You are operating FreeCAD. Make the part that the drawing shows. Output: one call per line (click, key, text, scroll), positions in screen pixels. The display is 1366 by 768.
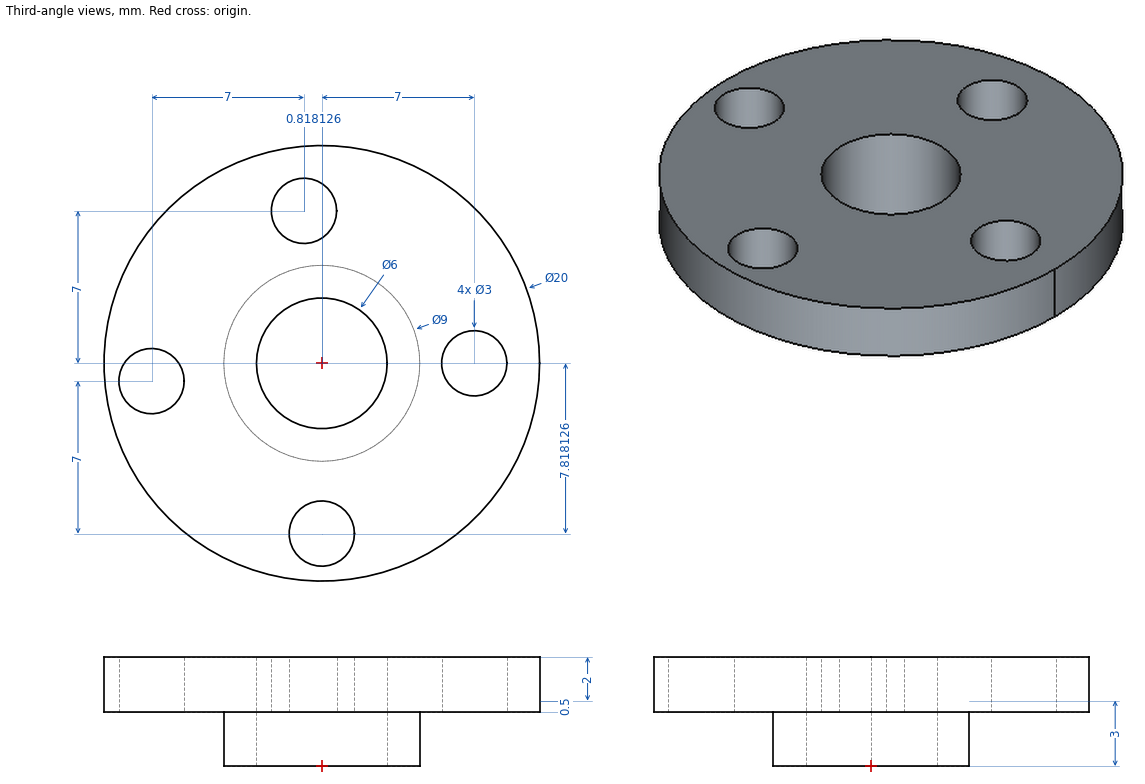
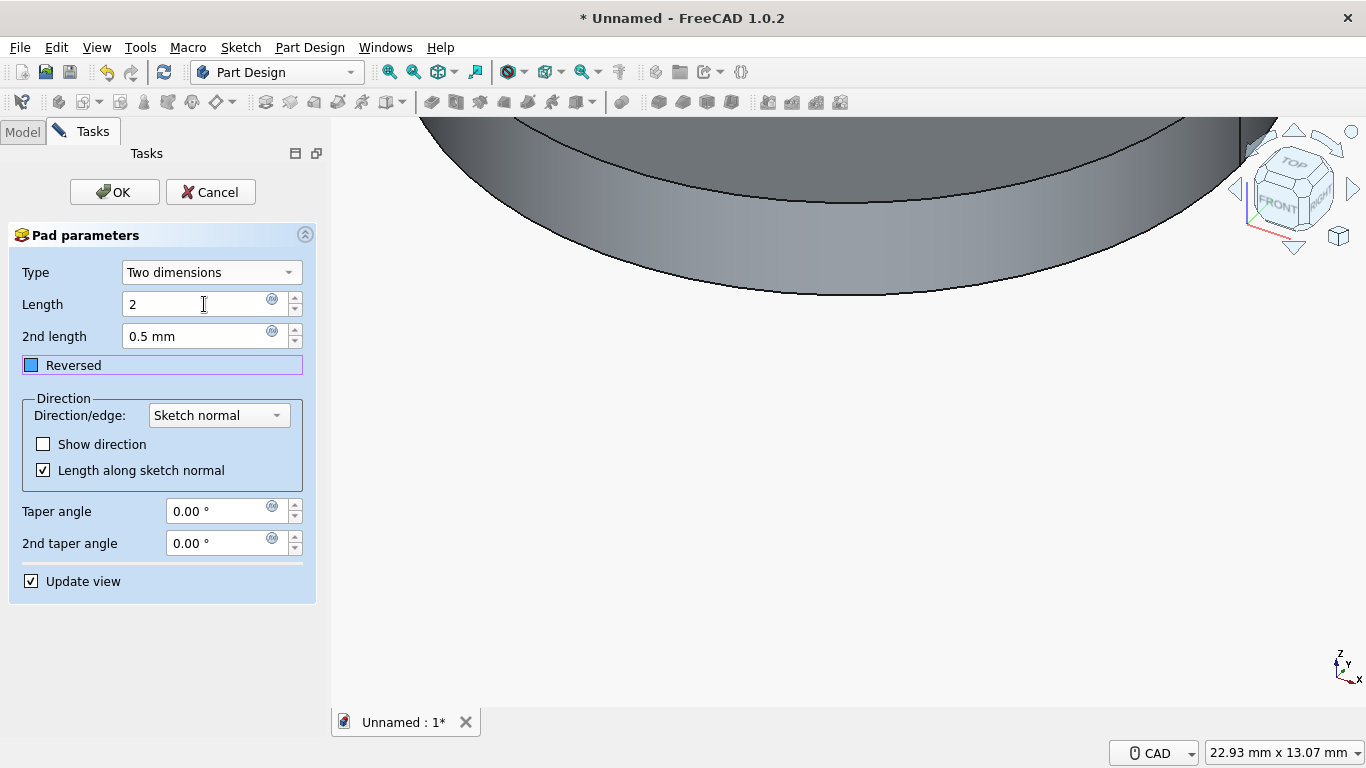
click(115, 192)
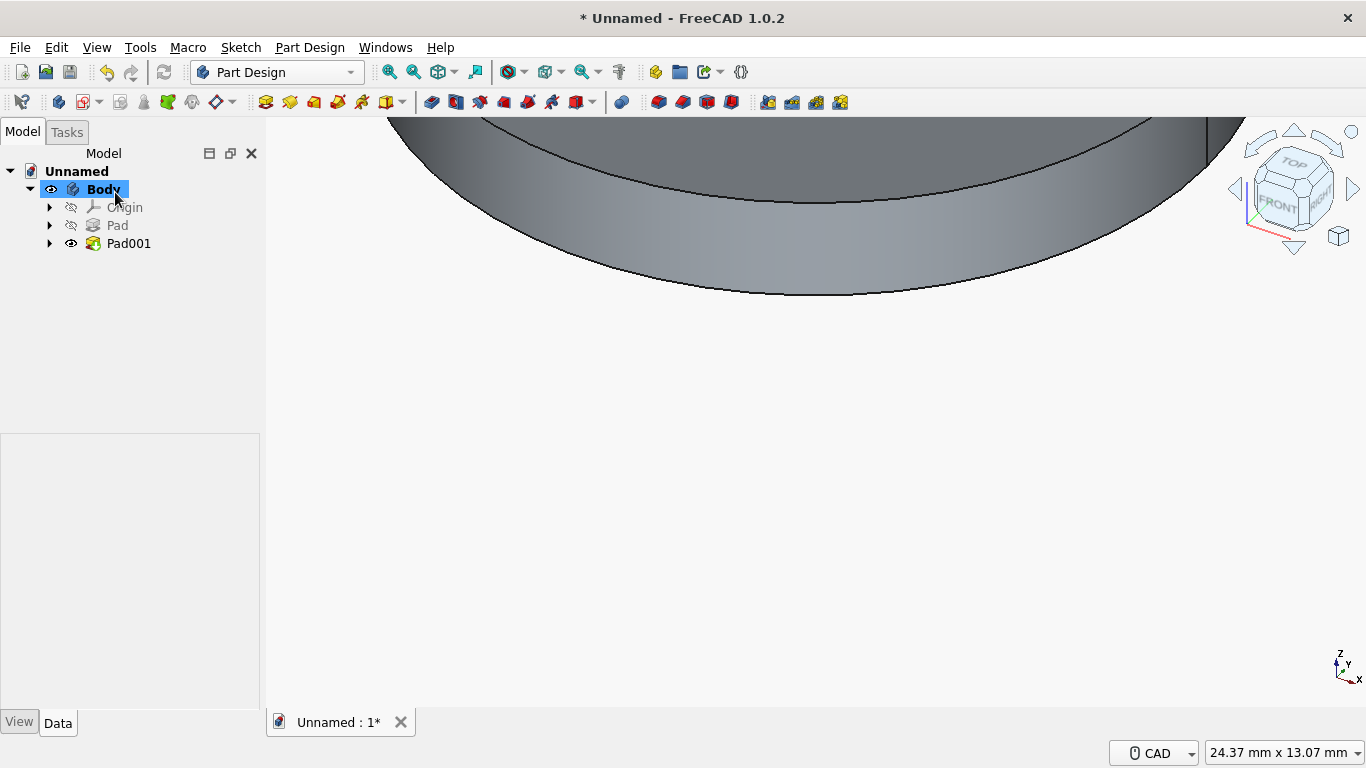
key(v)
key(f)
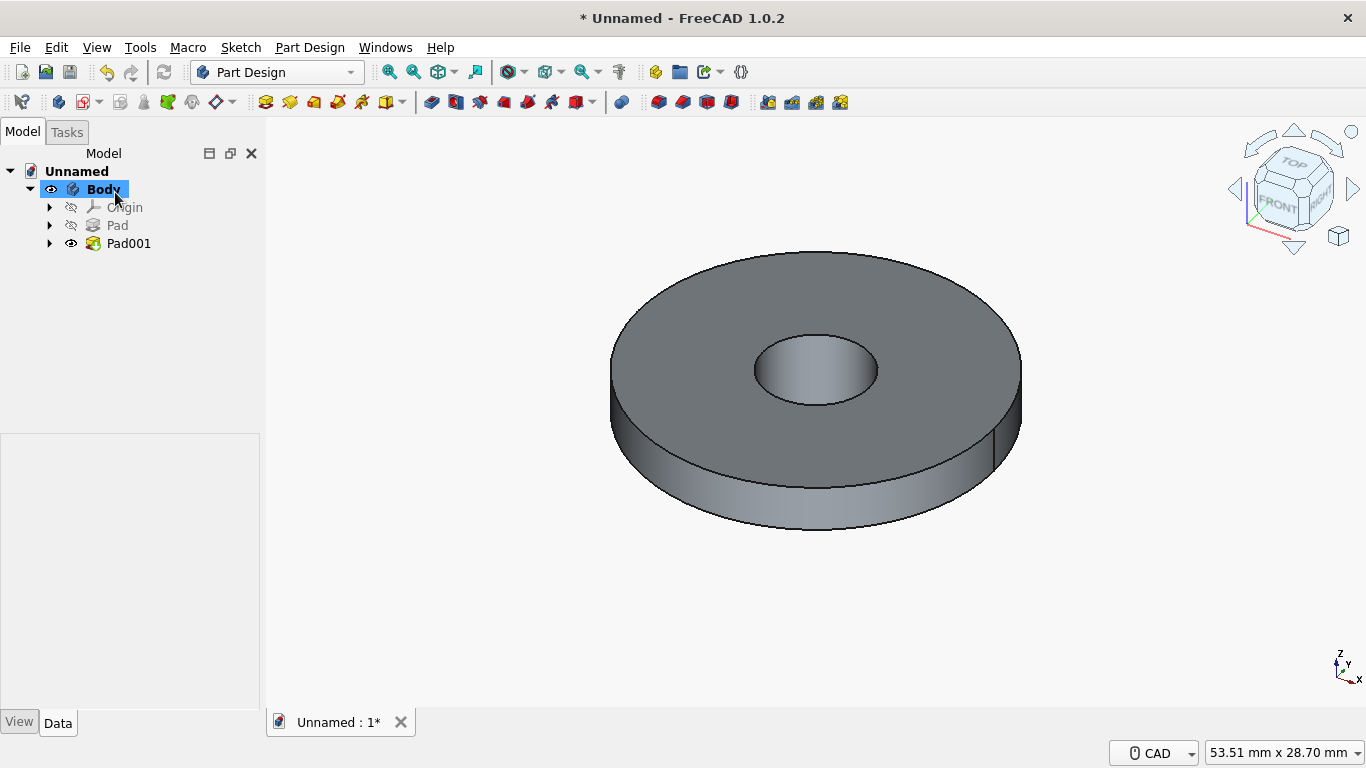
click(744, 306)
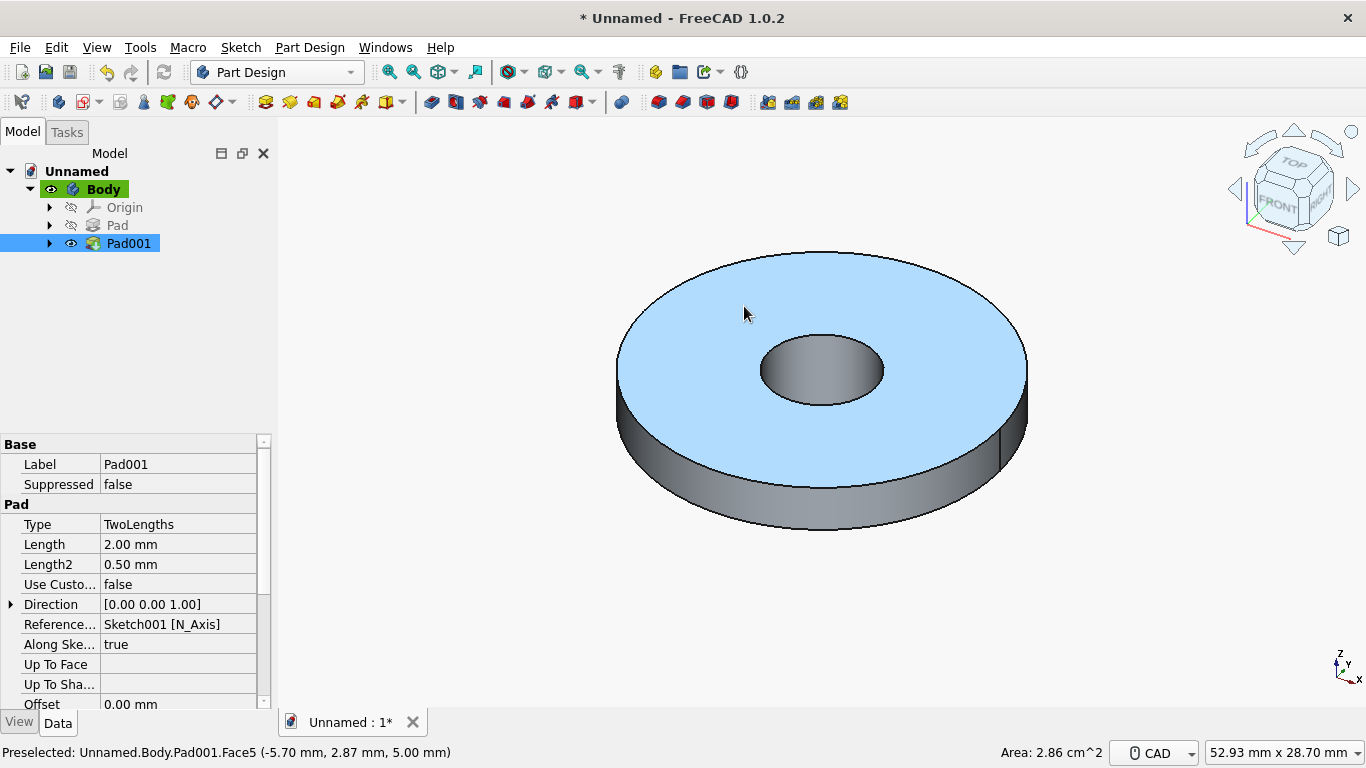
click(84, 102)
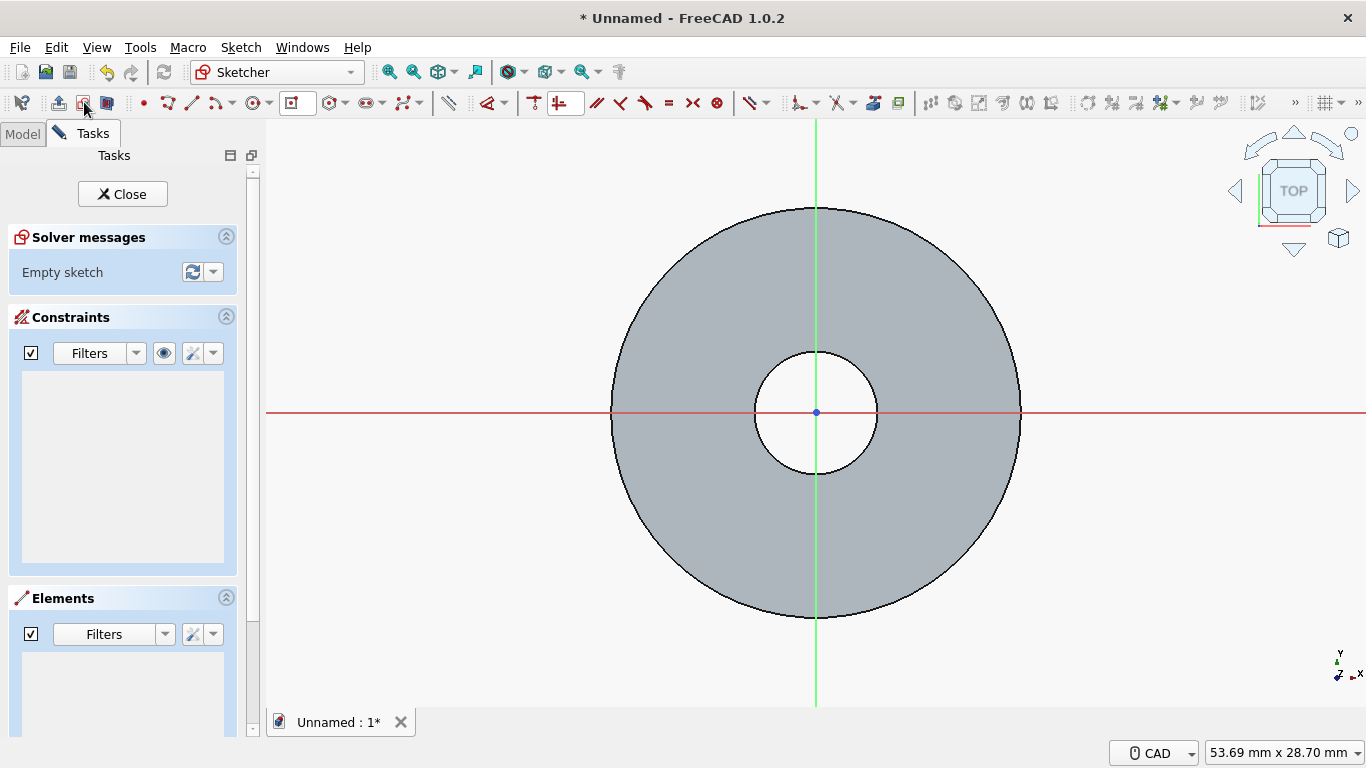
key(g)
key(c)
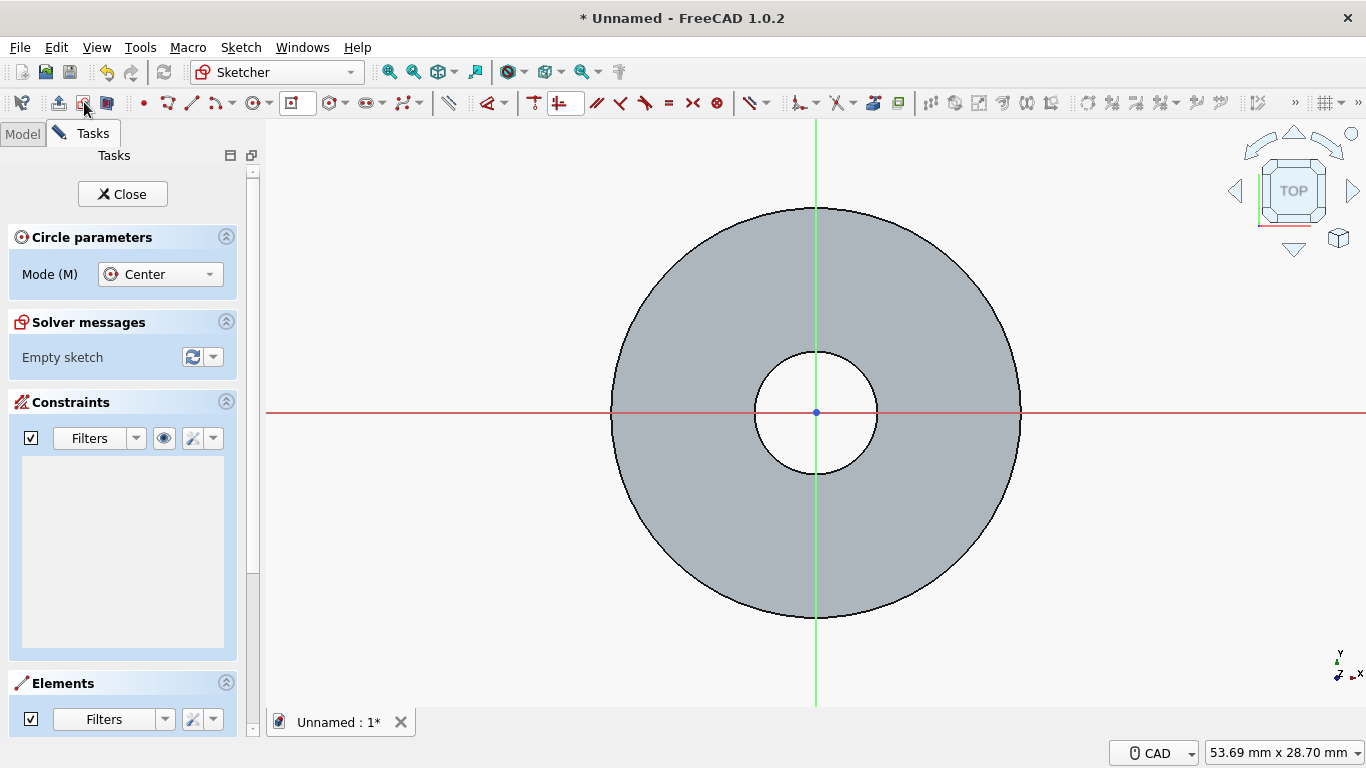
click(959, 413)
move(981, 391)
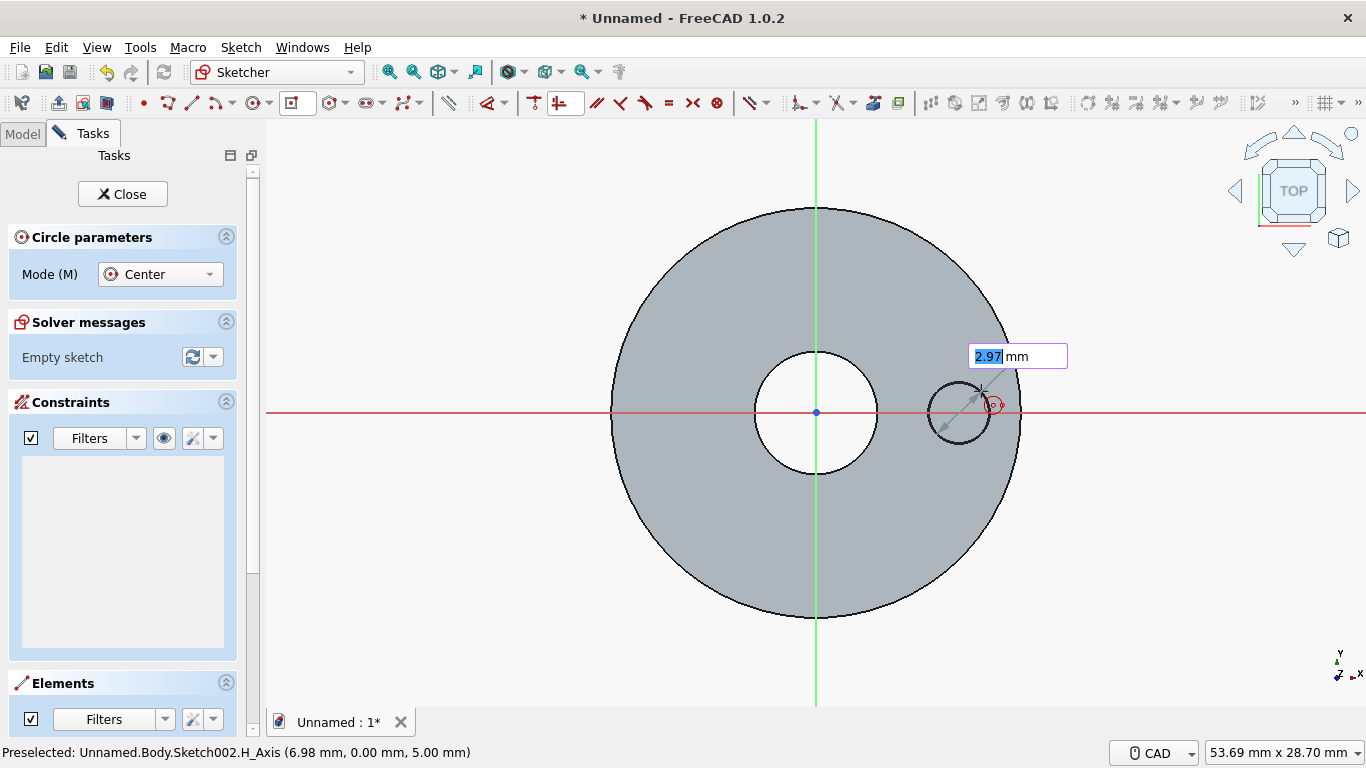
text(3)
key(Return)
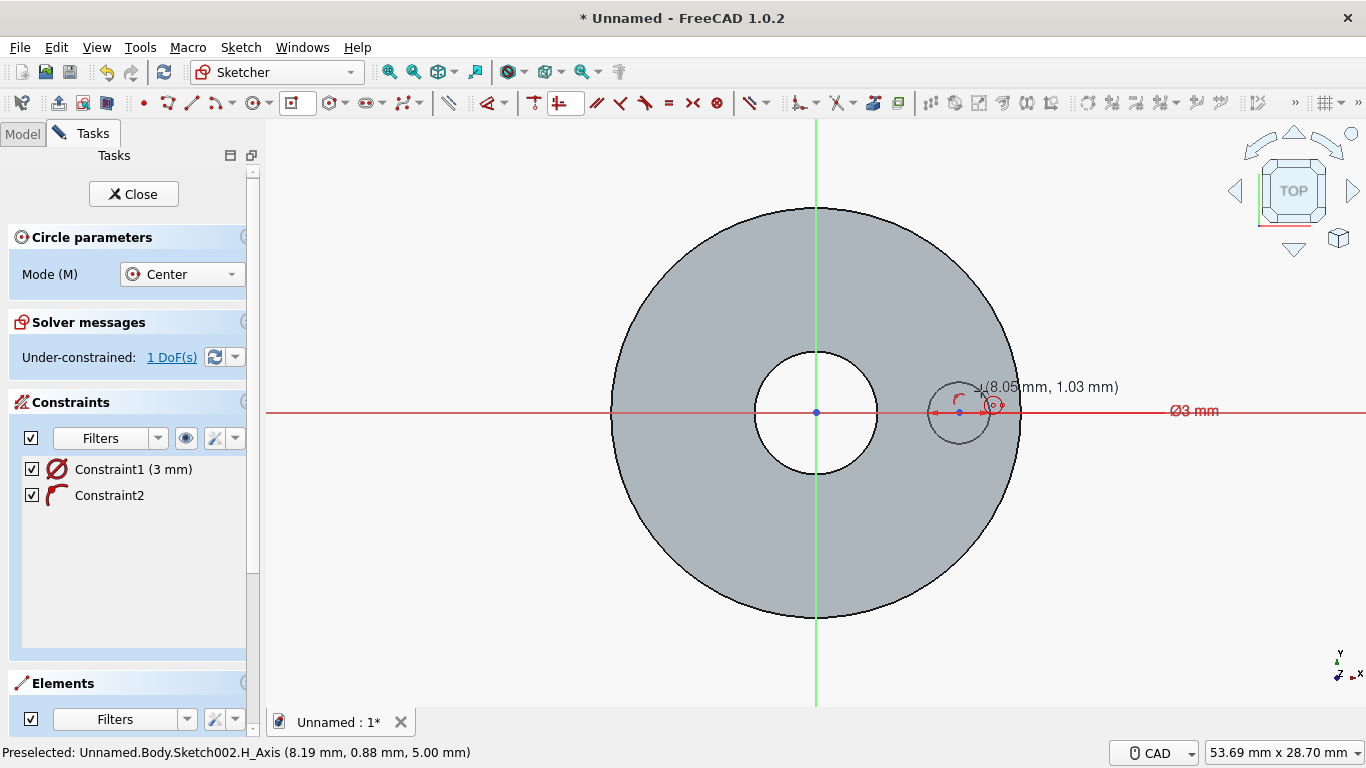
click(799, 270)
move(778, 248)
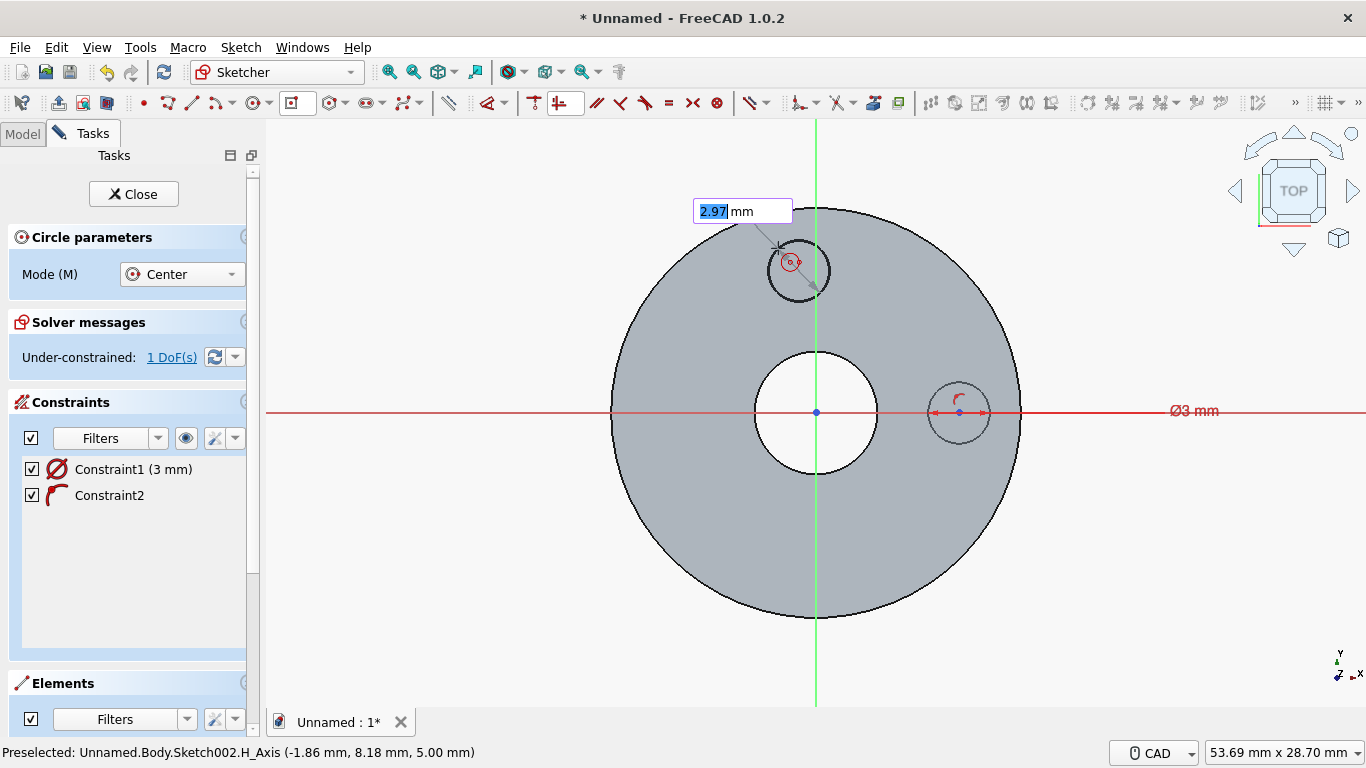
text(3)
key(Return)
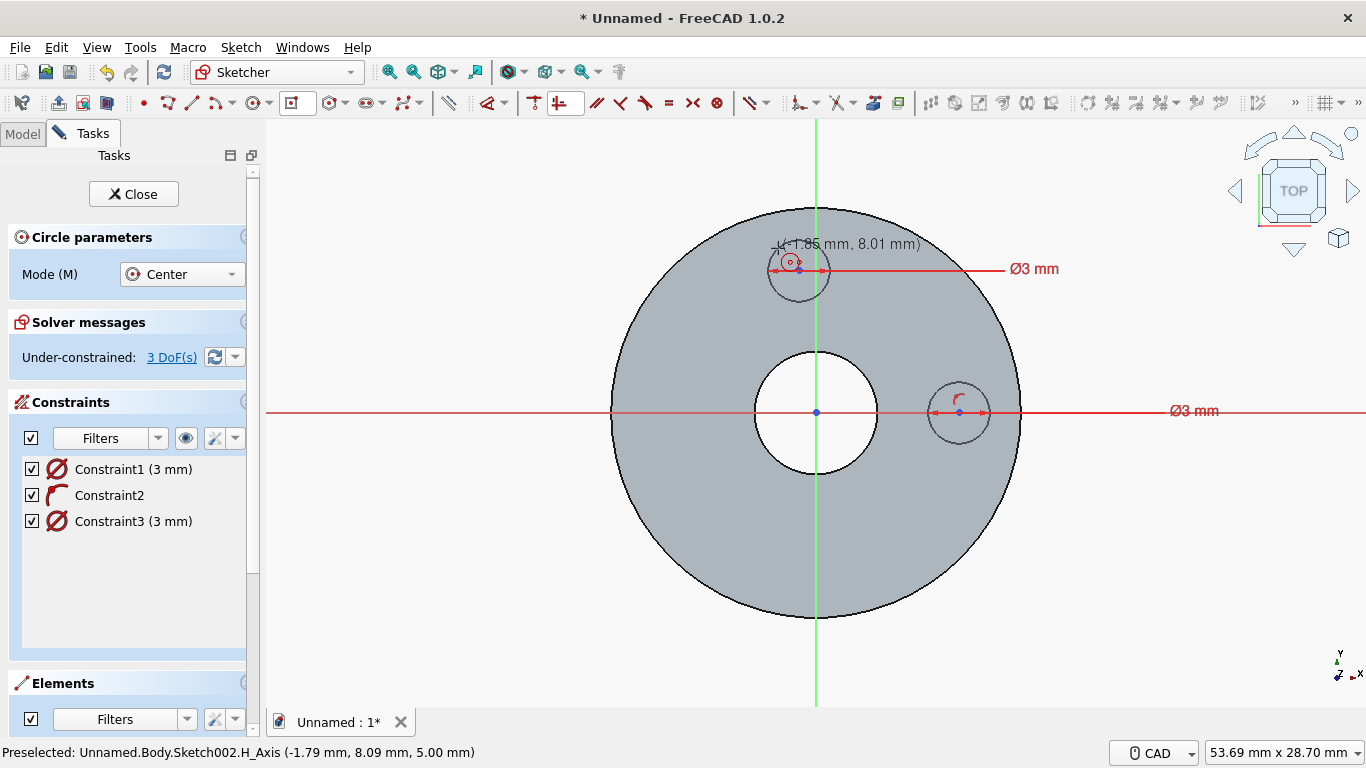
click(816, 573)
move(838, 551)